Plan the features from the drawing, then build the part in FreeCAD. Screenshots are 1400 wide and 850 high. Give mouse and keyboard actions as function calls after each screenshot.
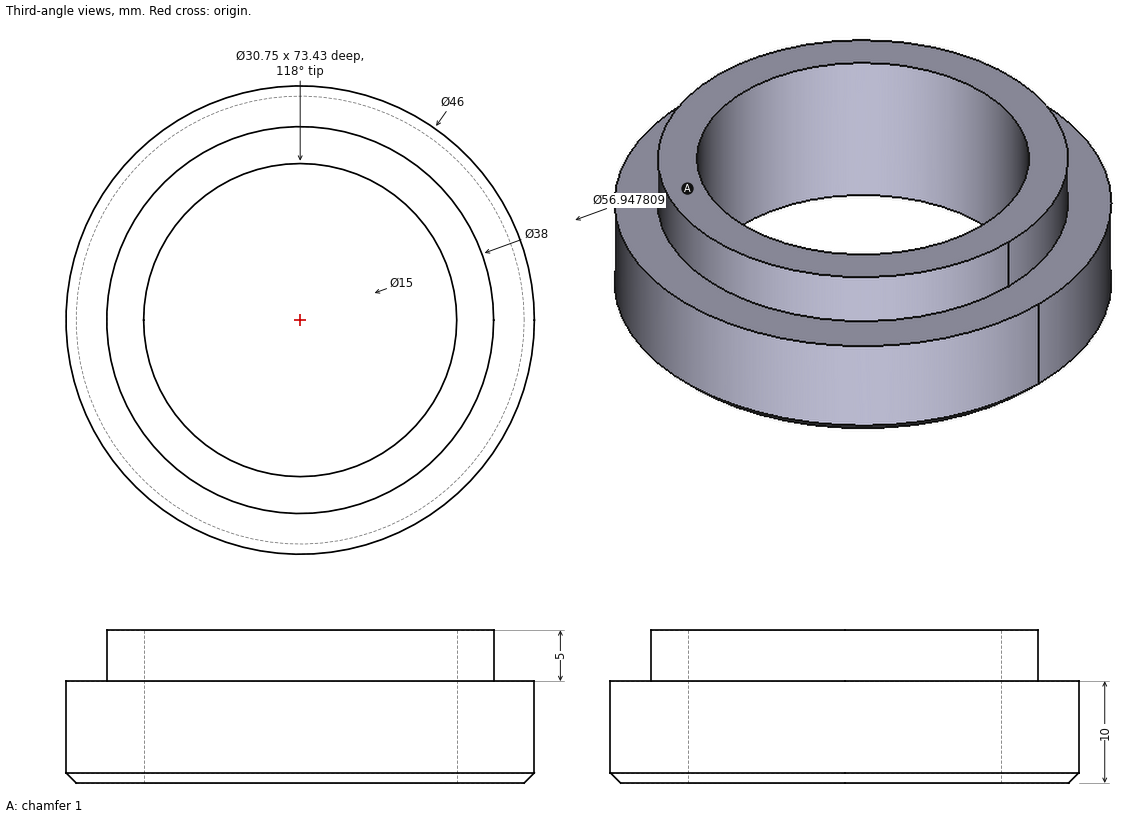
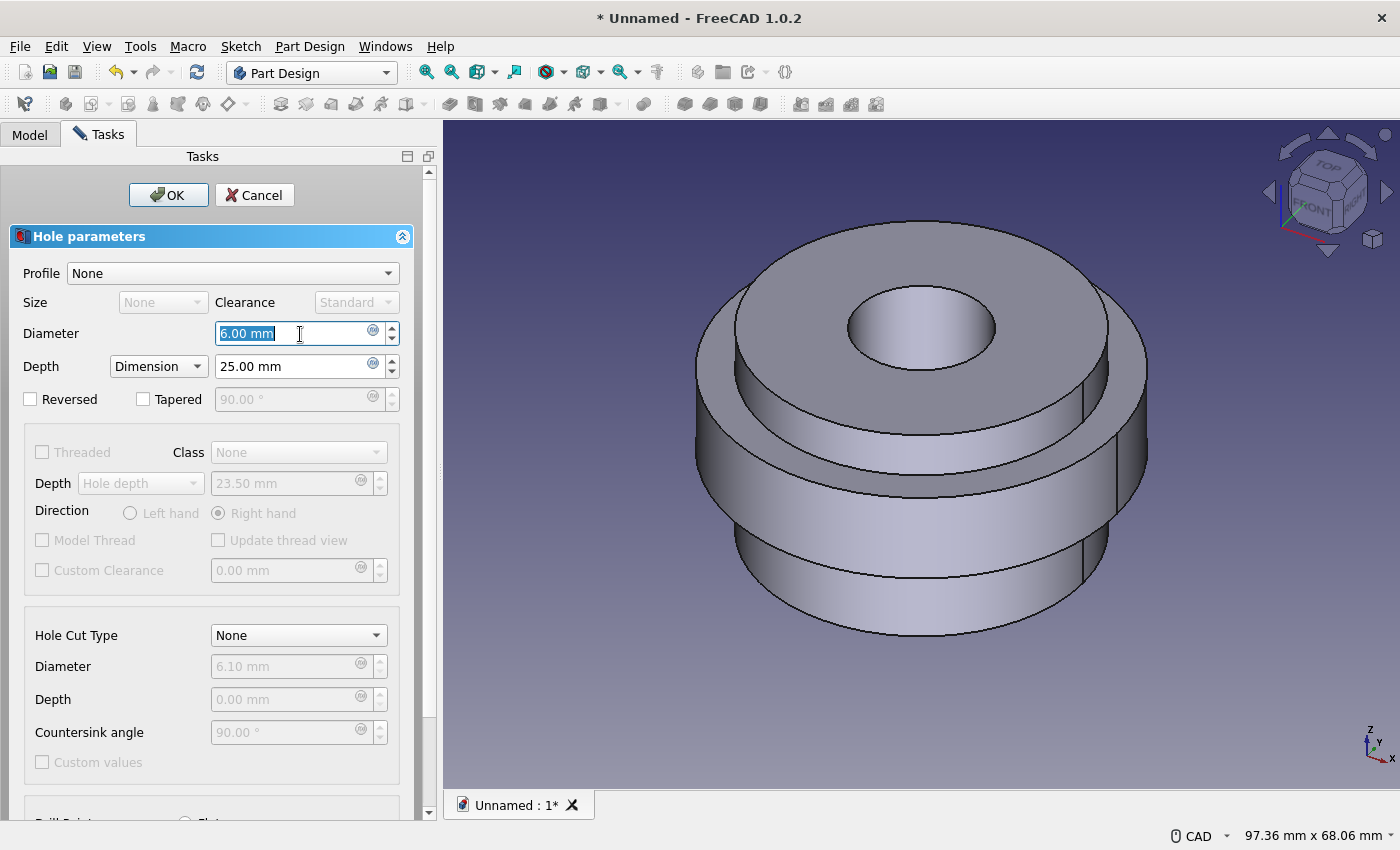
text(30.75)
key(Tab)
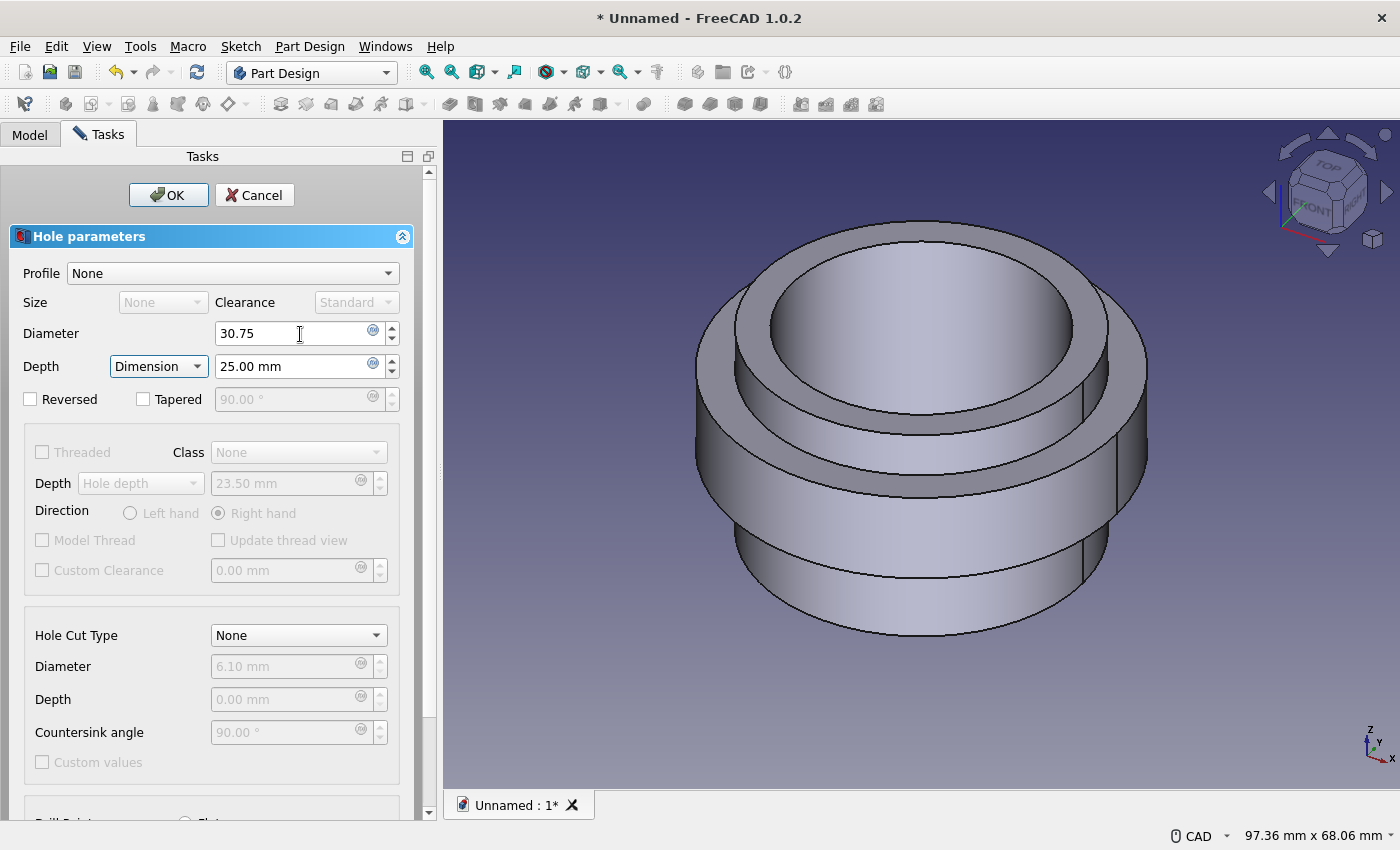
triple_click(300, 366)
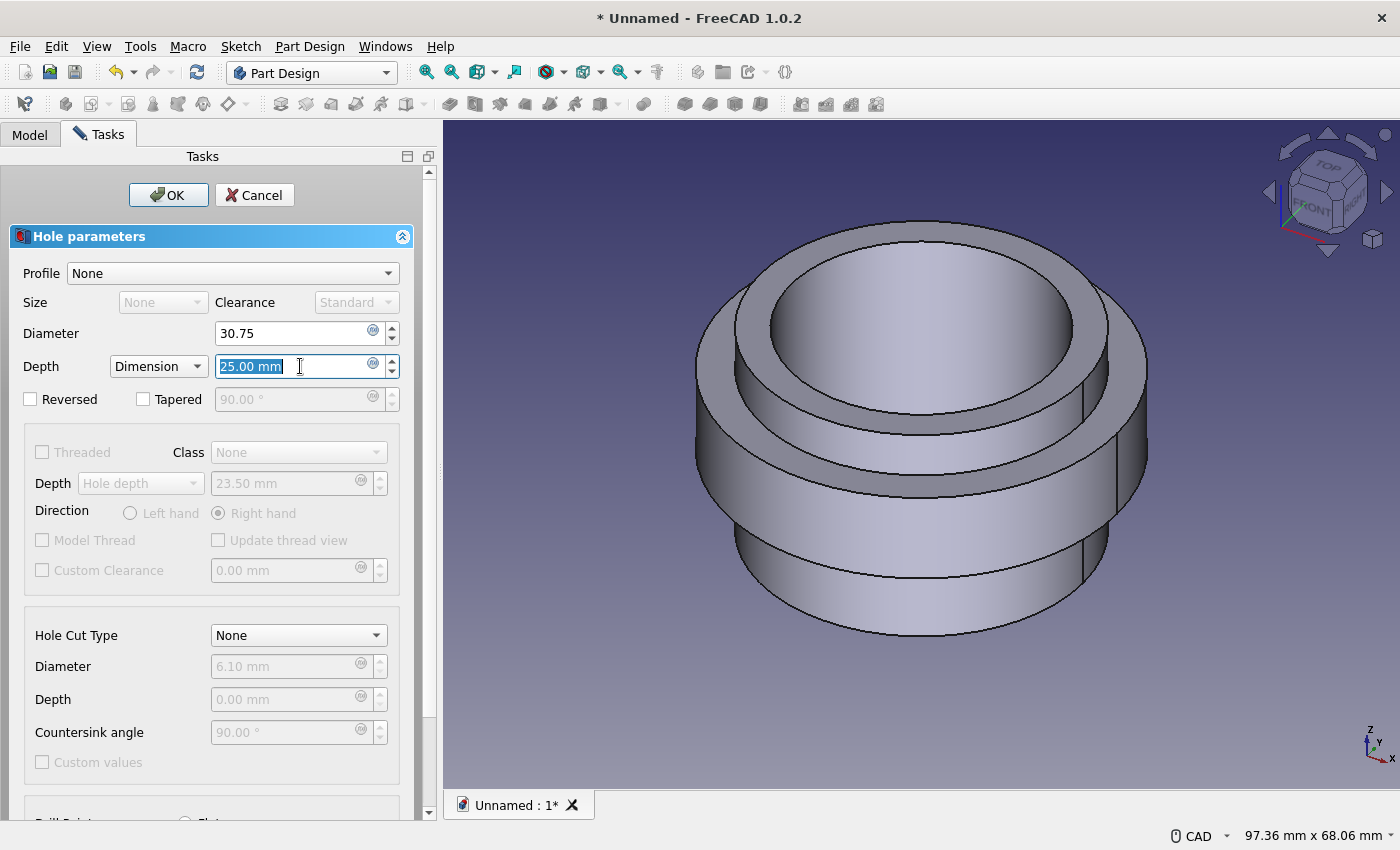
text(73.43)
key(Tab)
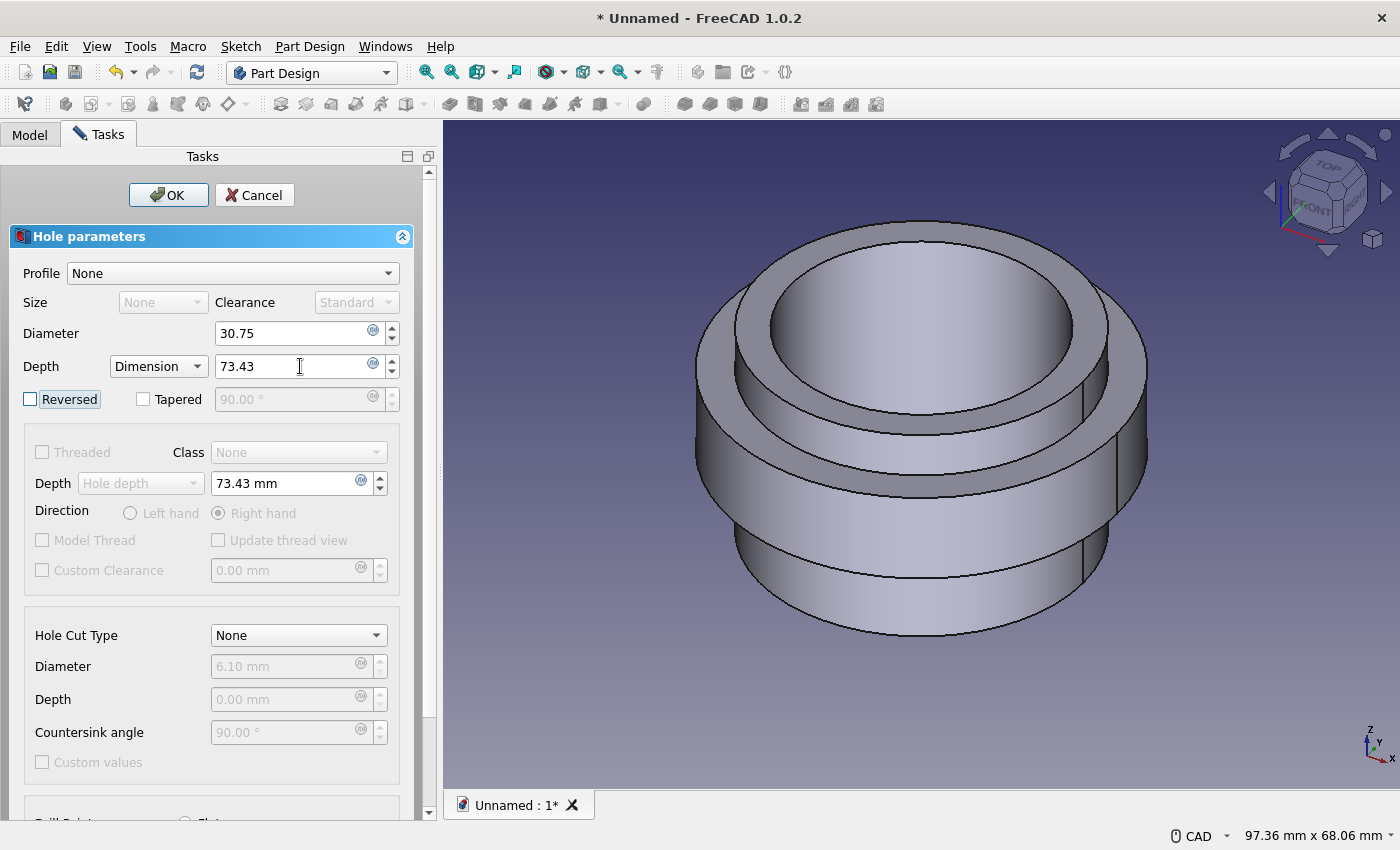
click(169, 195)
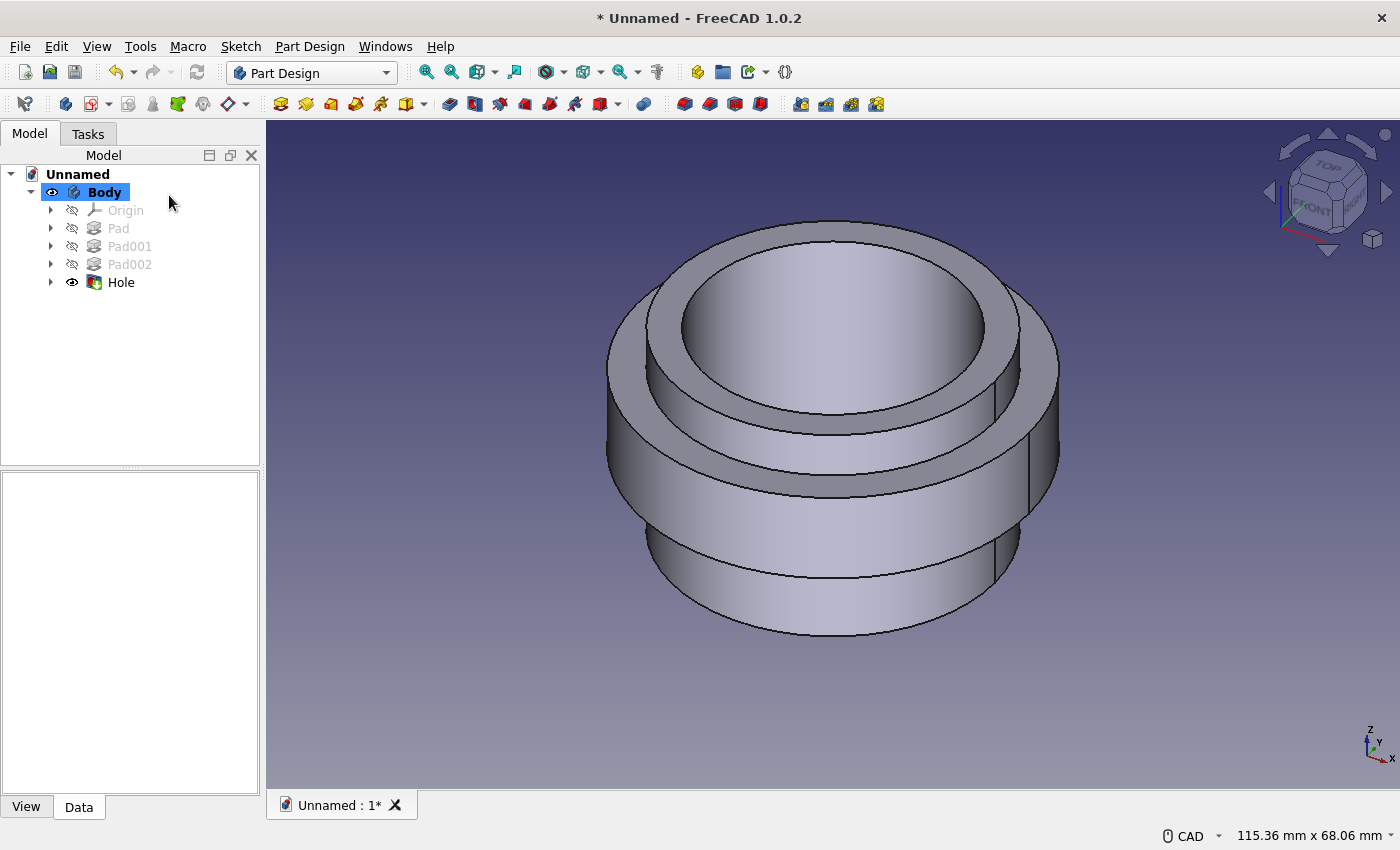
key(5)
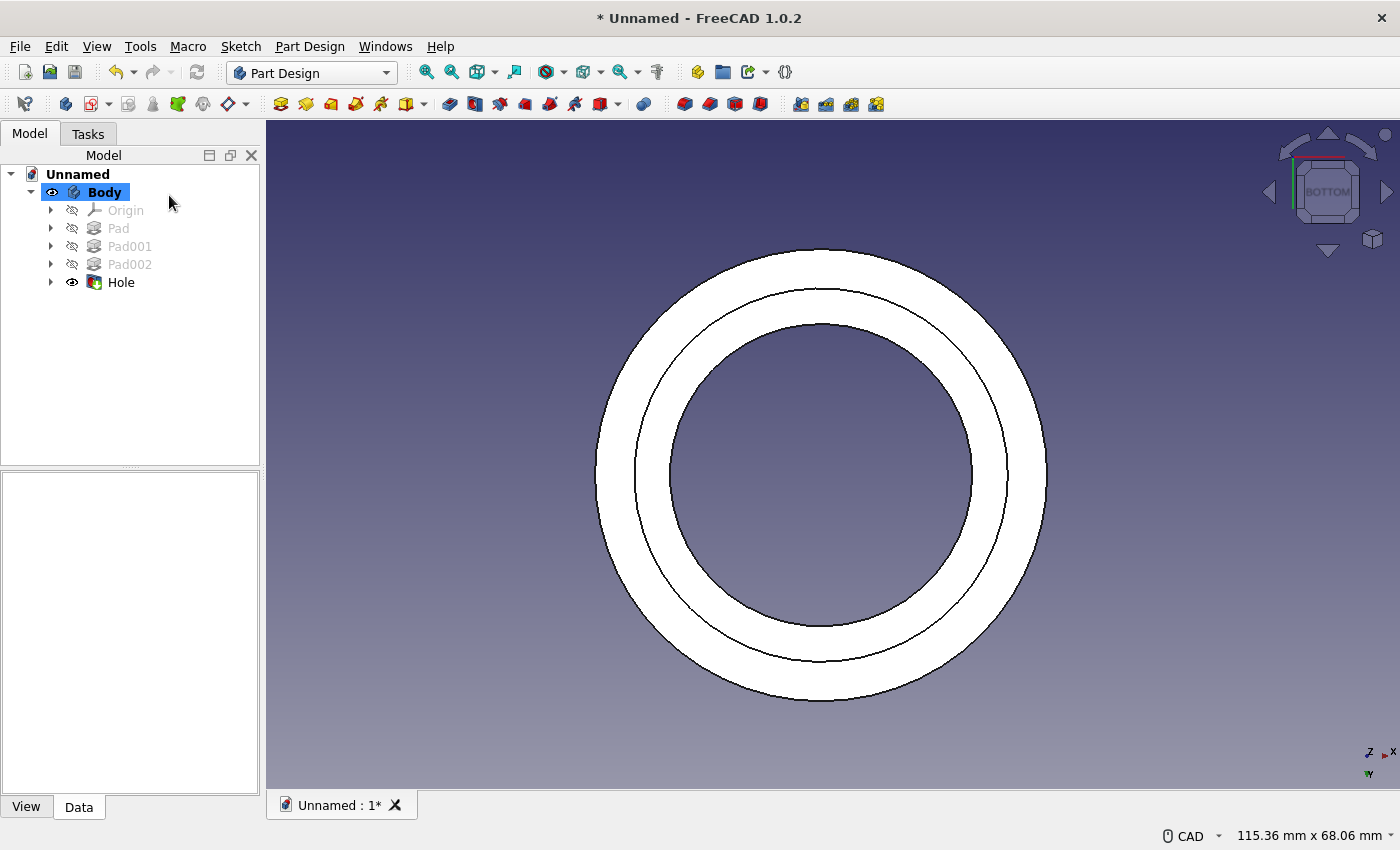
click(768, 634)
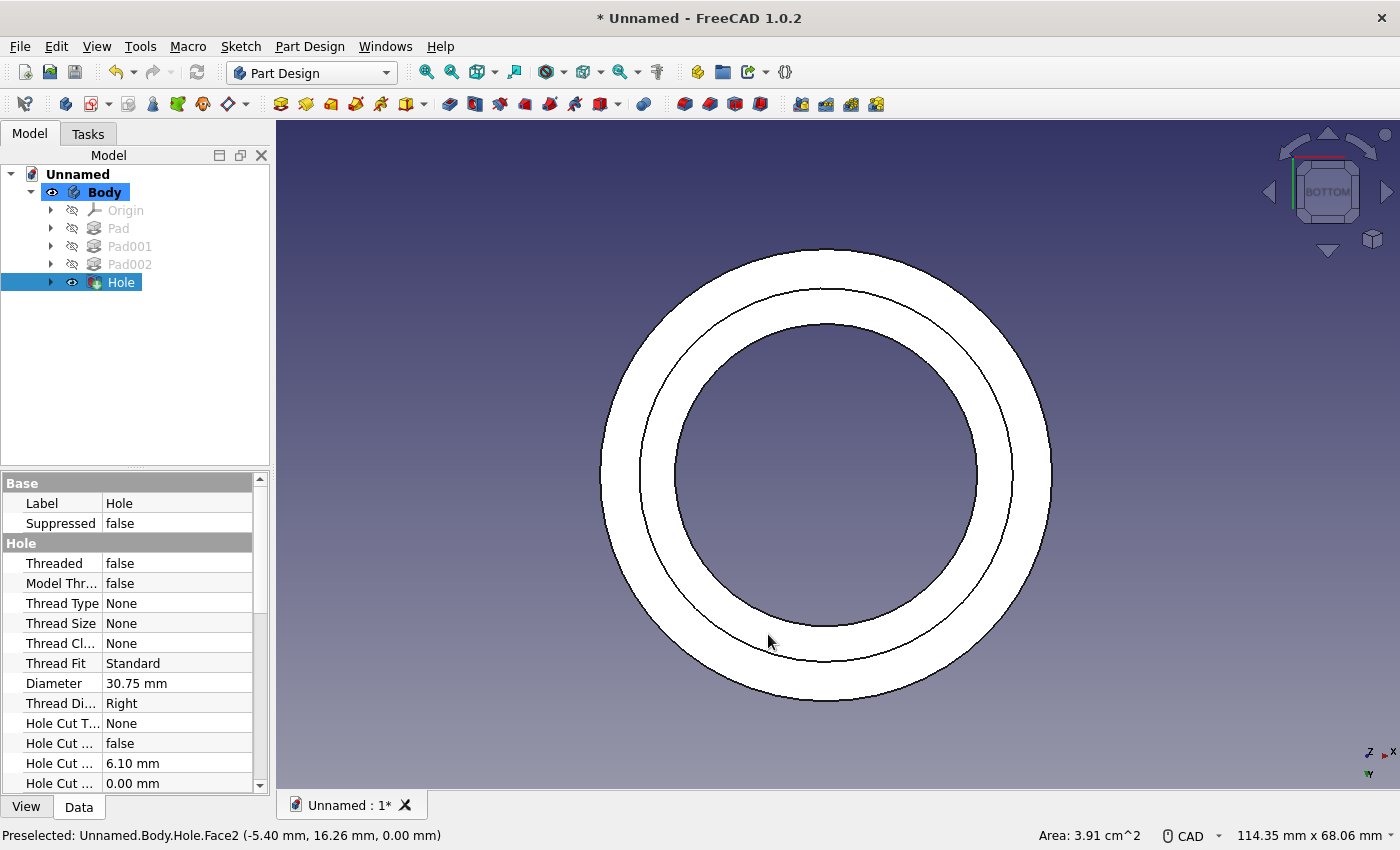
click(90, 104)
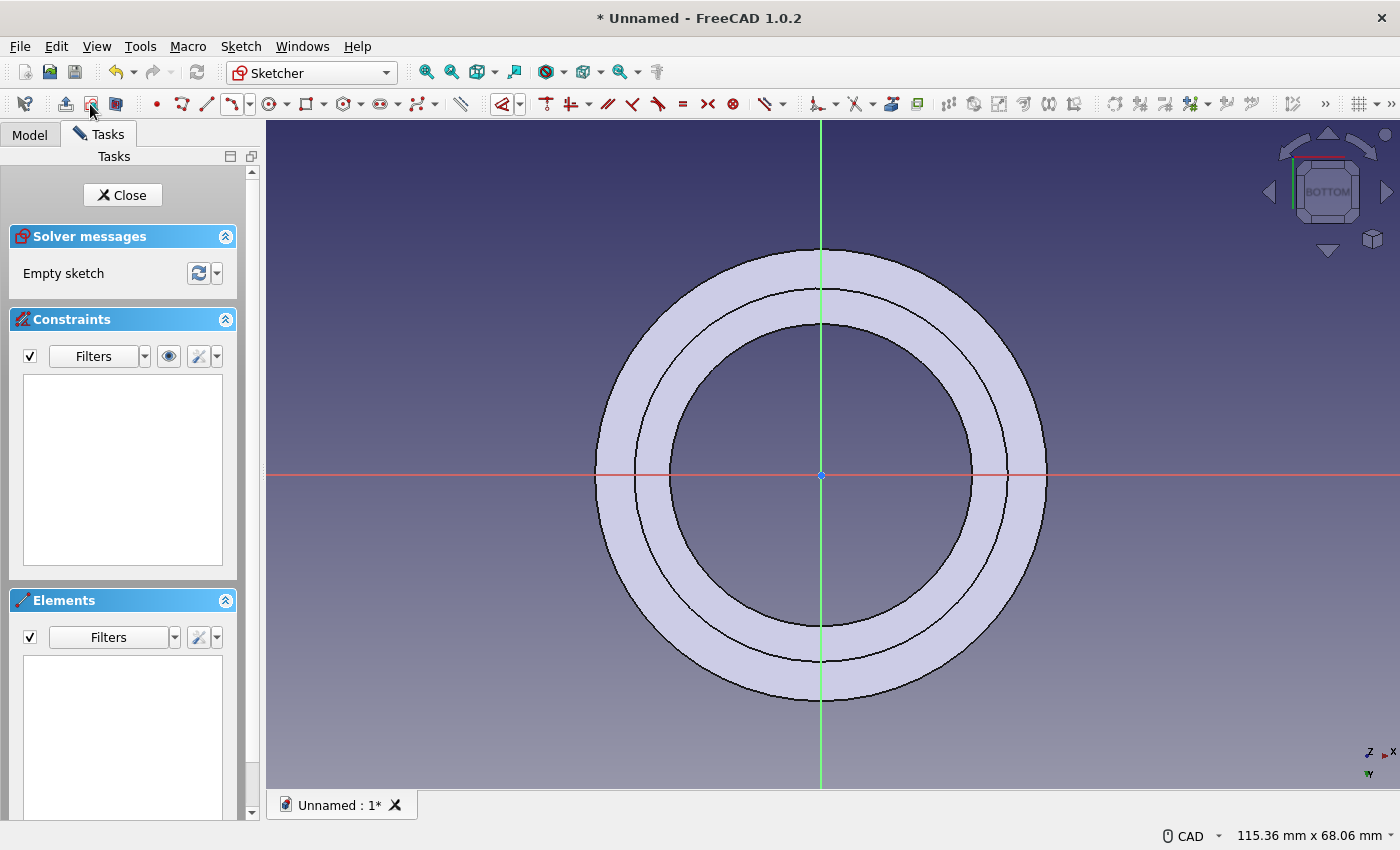
scroll(509, 361, down, 1)